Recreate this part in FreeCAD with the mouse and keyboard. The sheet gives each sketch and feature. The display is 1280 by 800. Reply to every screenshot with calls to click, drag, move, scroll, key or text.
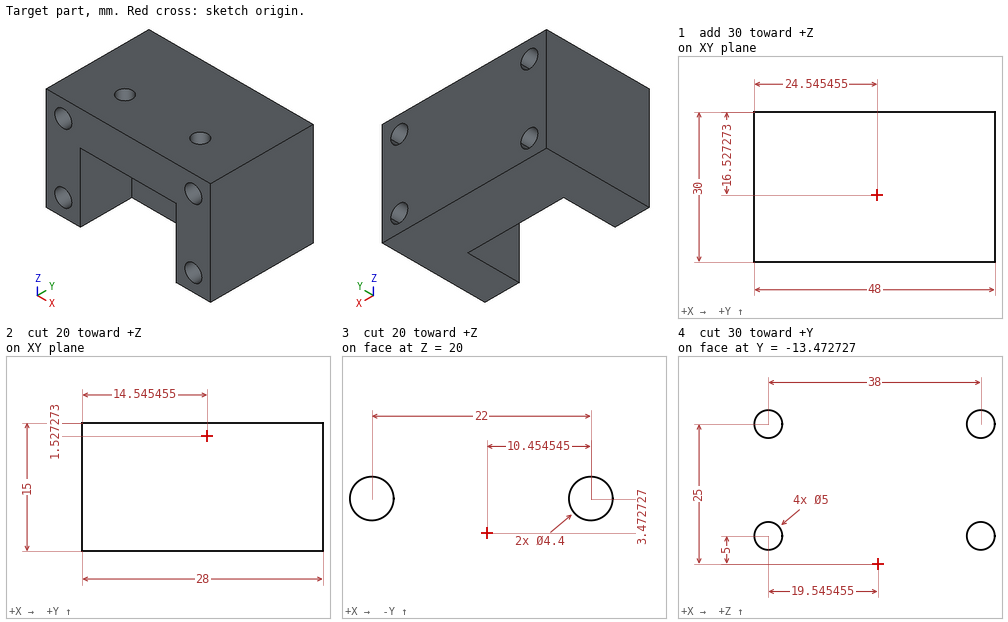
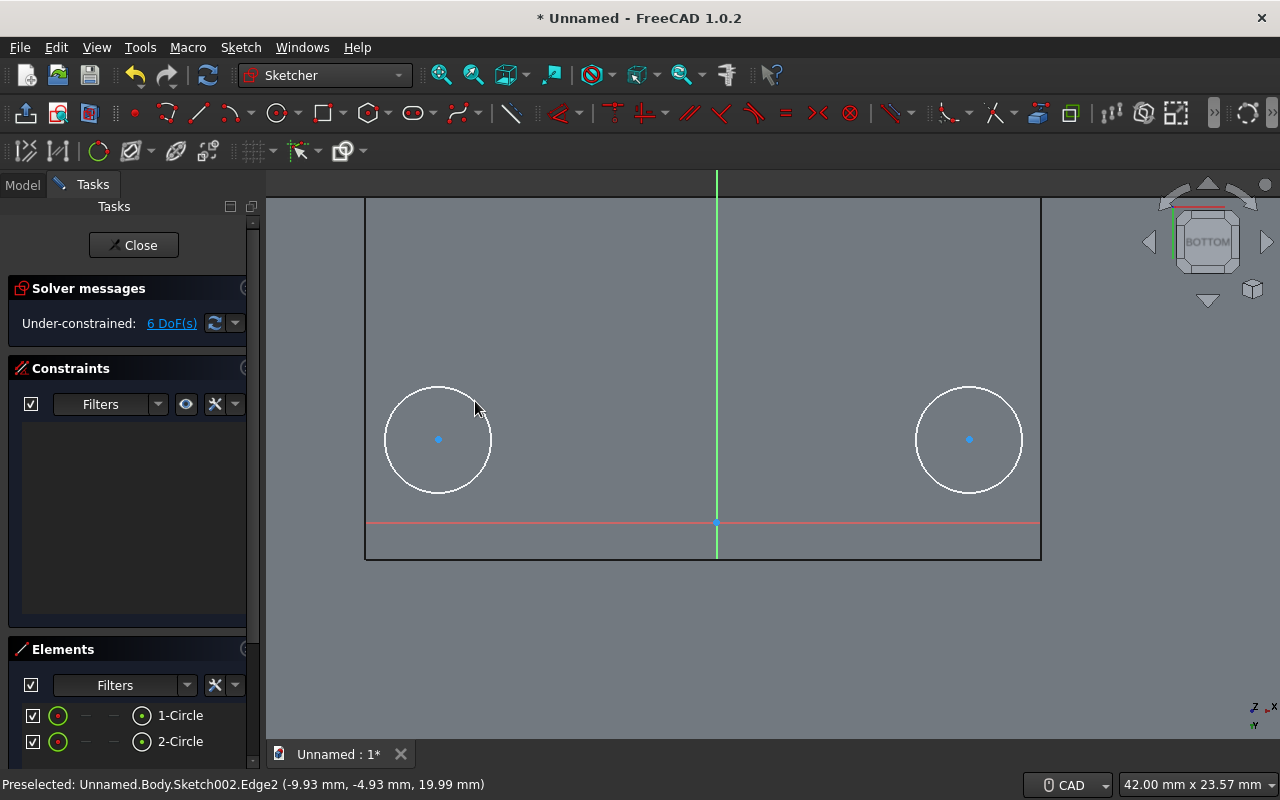
click(1006, 402)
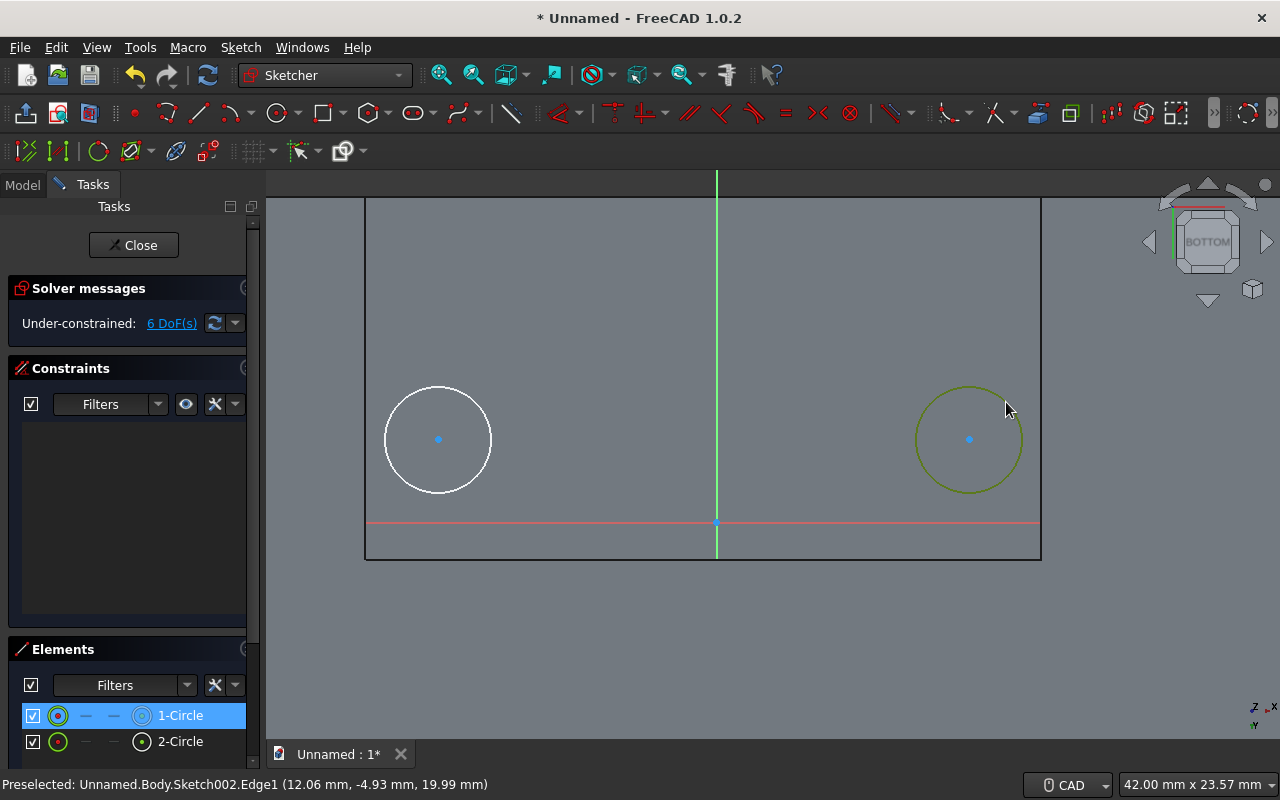
click(475, 402)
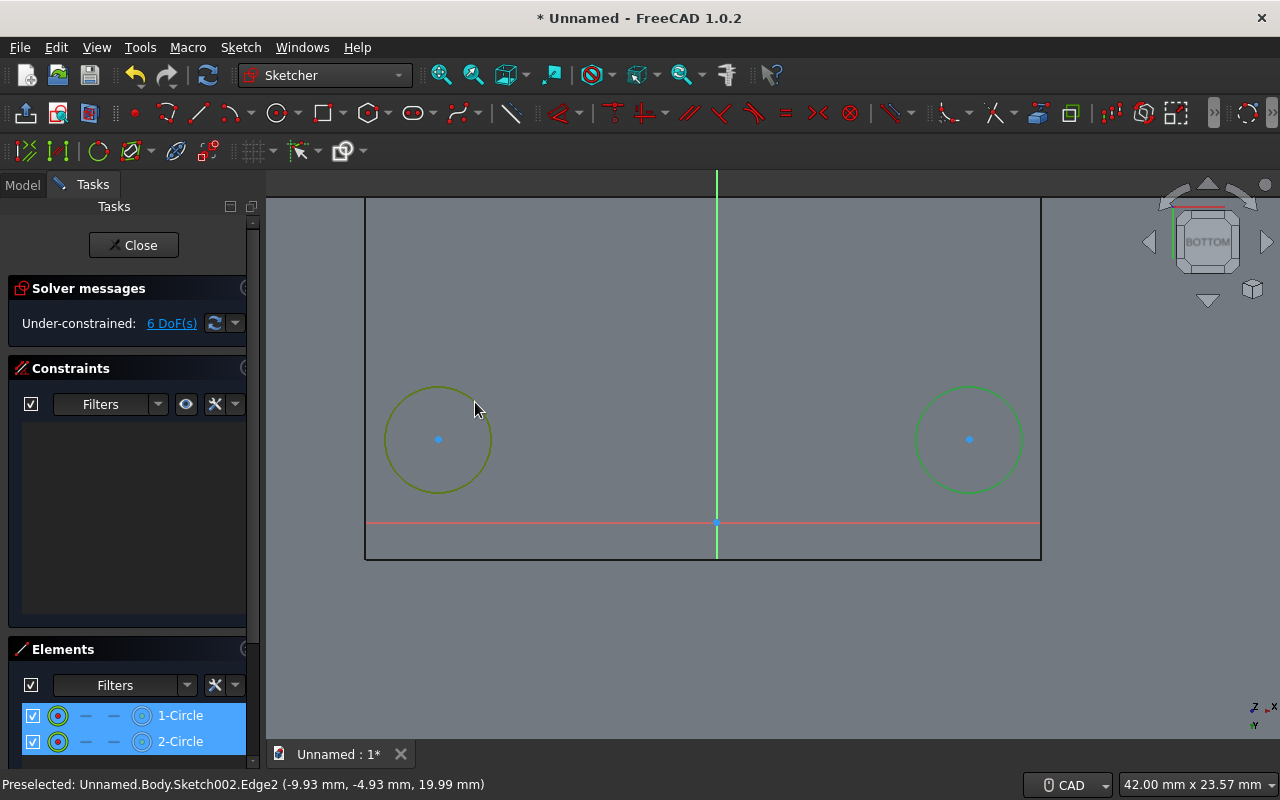
key(e)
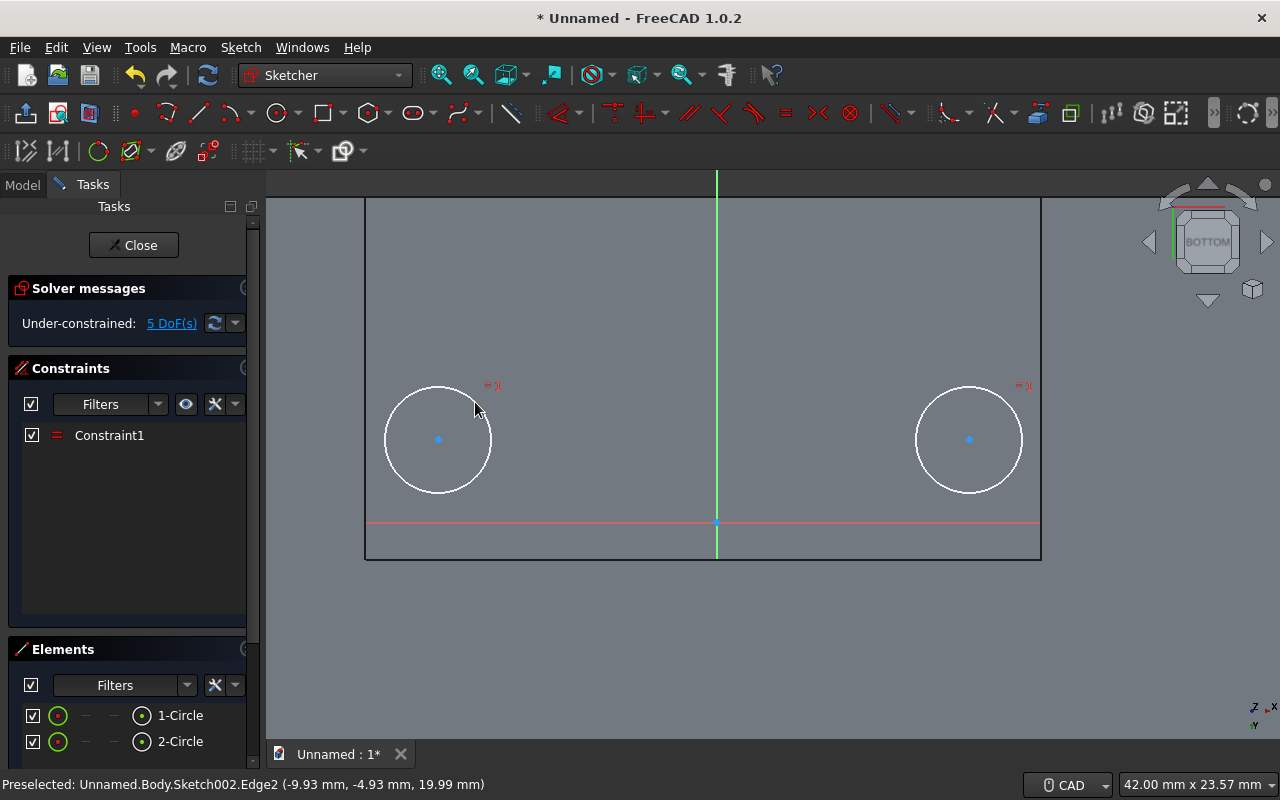
click(969, 440)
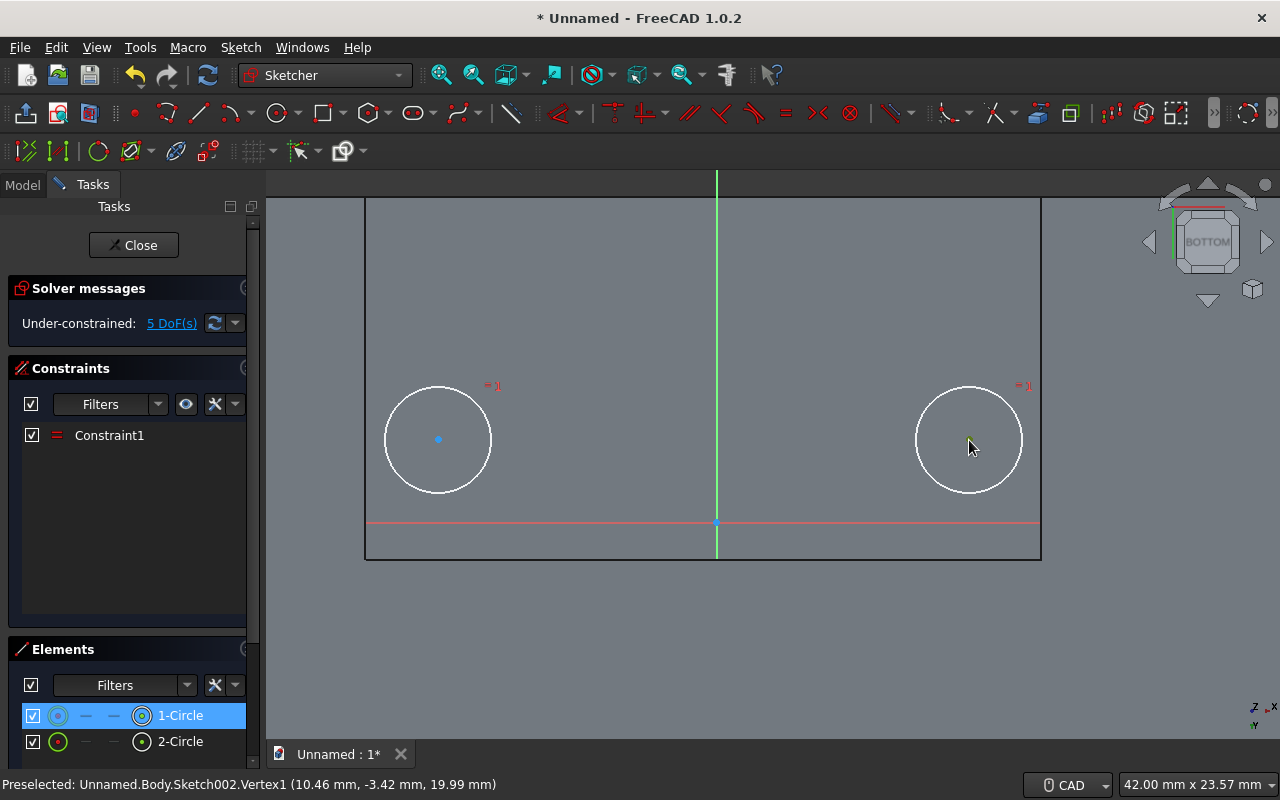
click(438, 440)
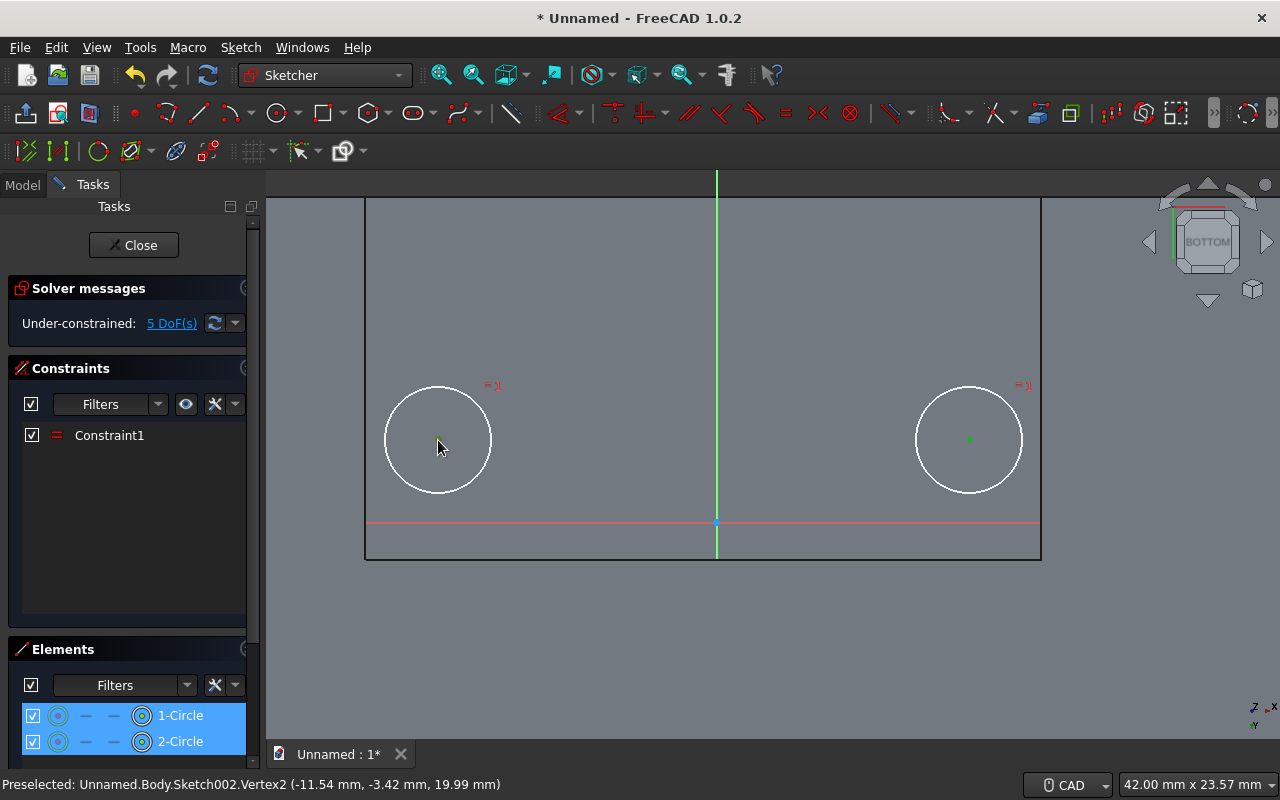
key(h)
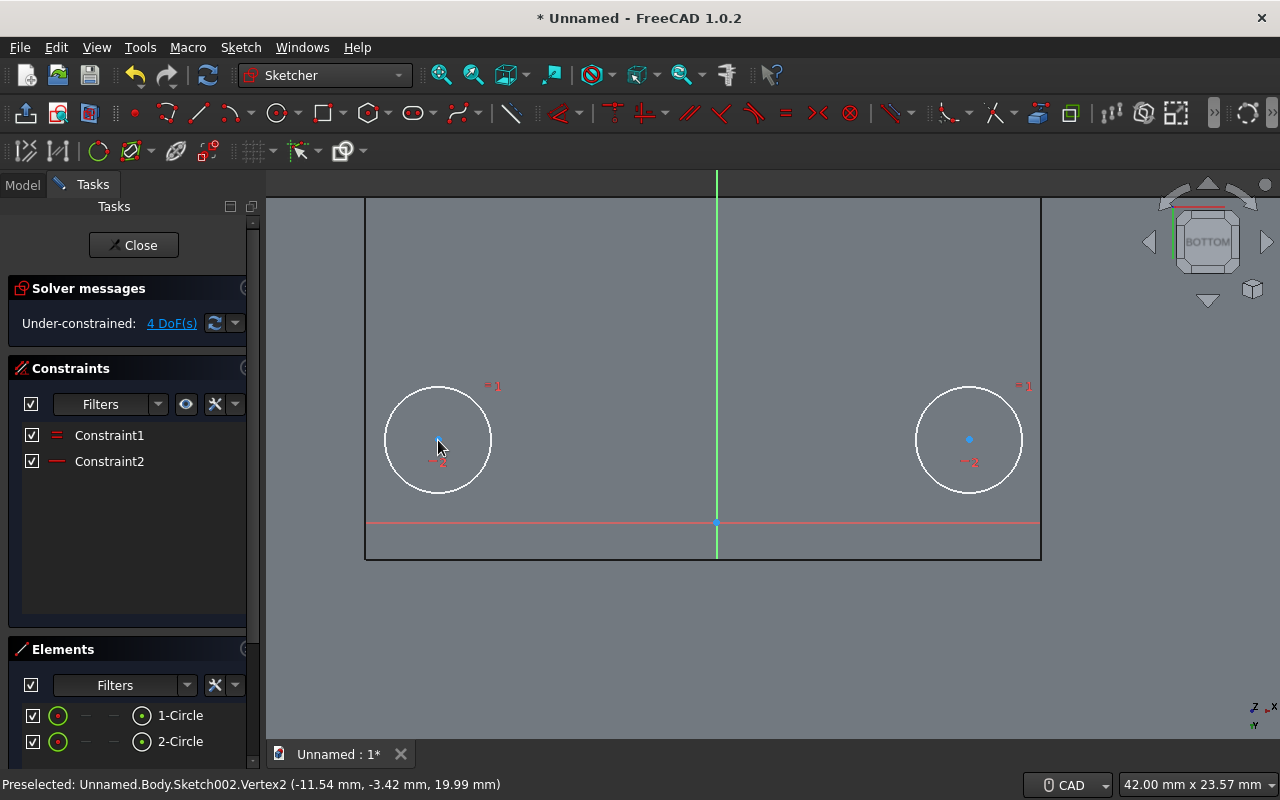
key(d)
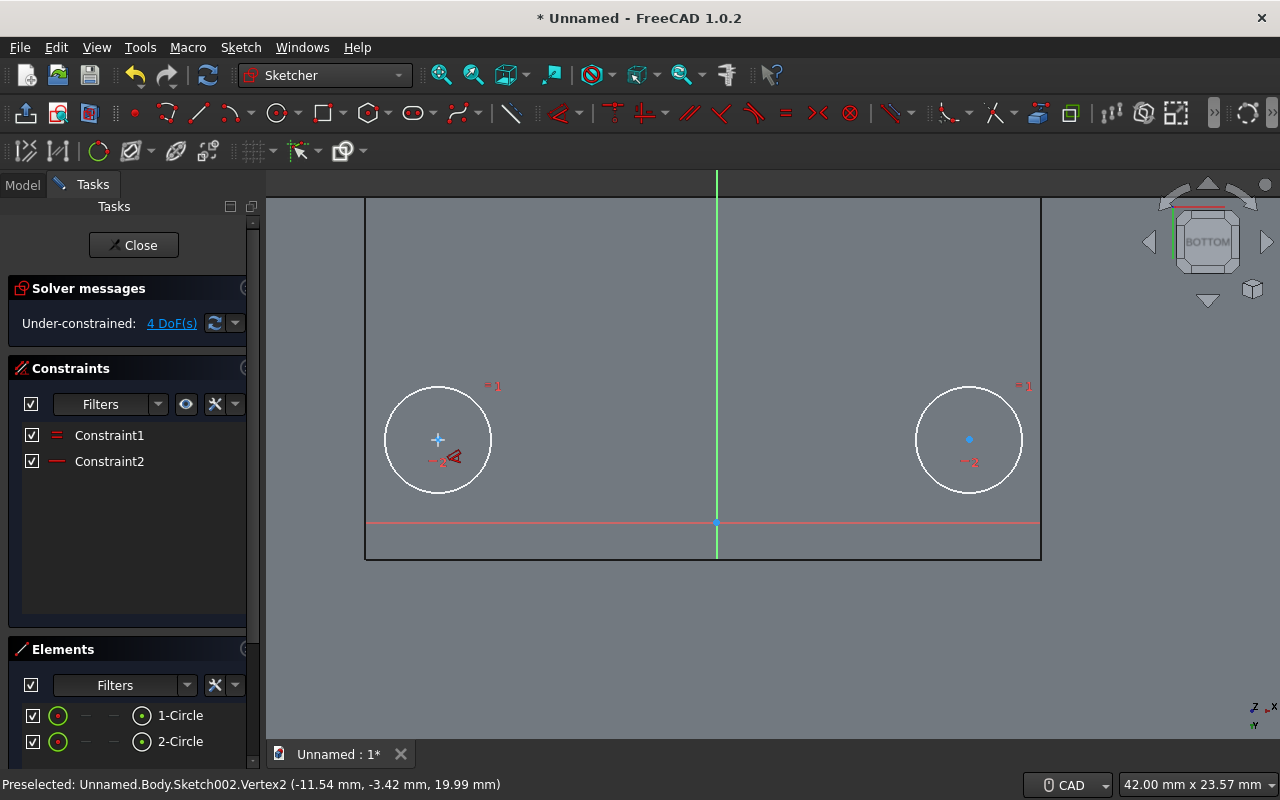
click(1006, 402)
click(1028, 379)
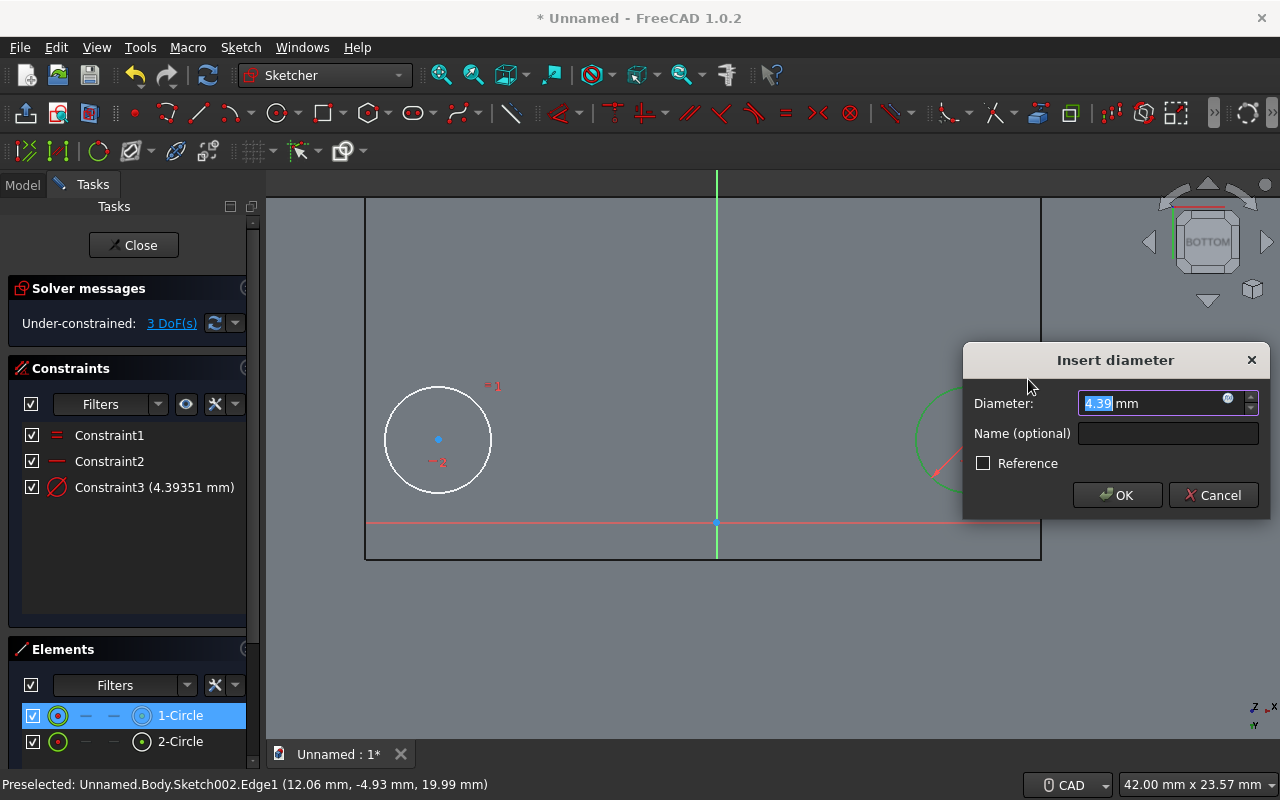
text(4.4)
key(Return)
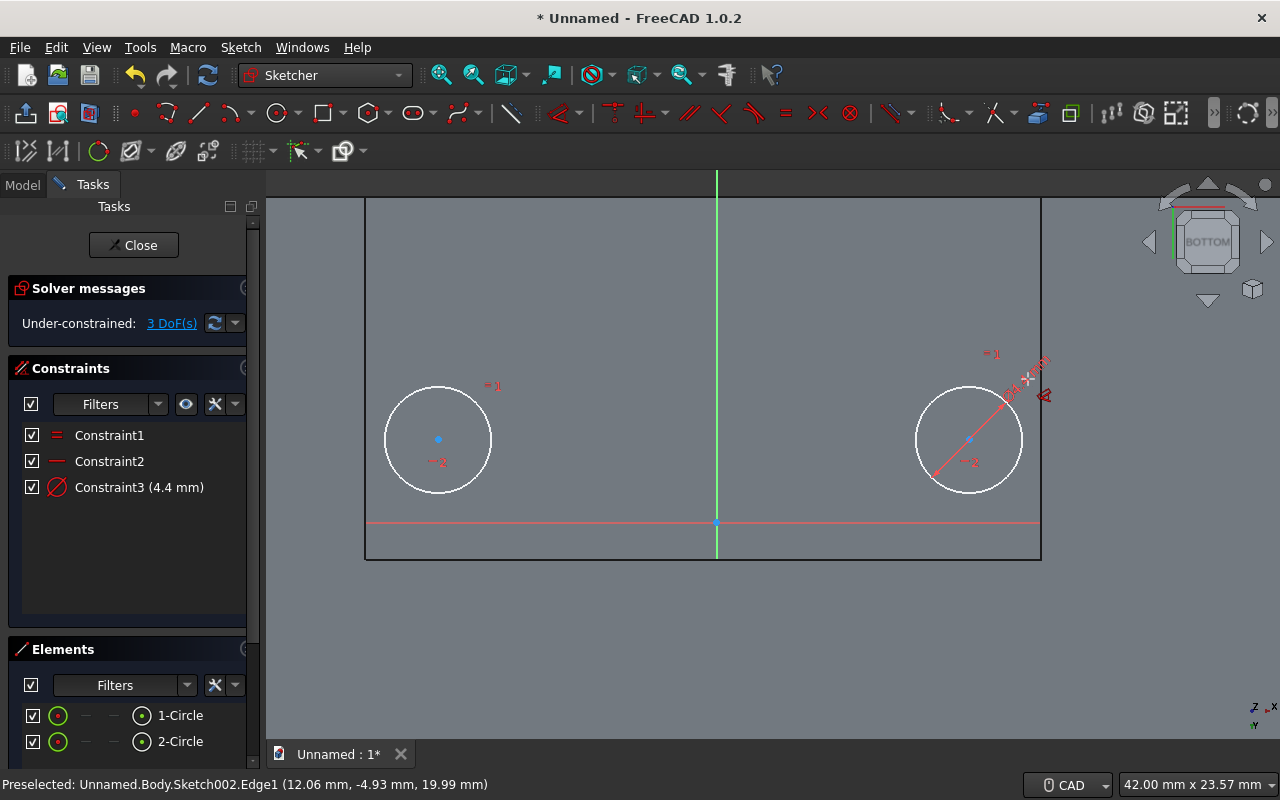
click(969, 440)